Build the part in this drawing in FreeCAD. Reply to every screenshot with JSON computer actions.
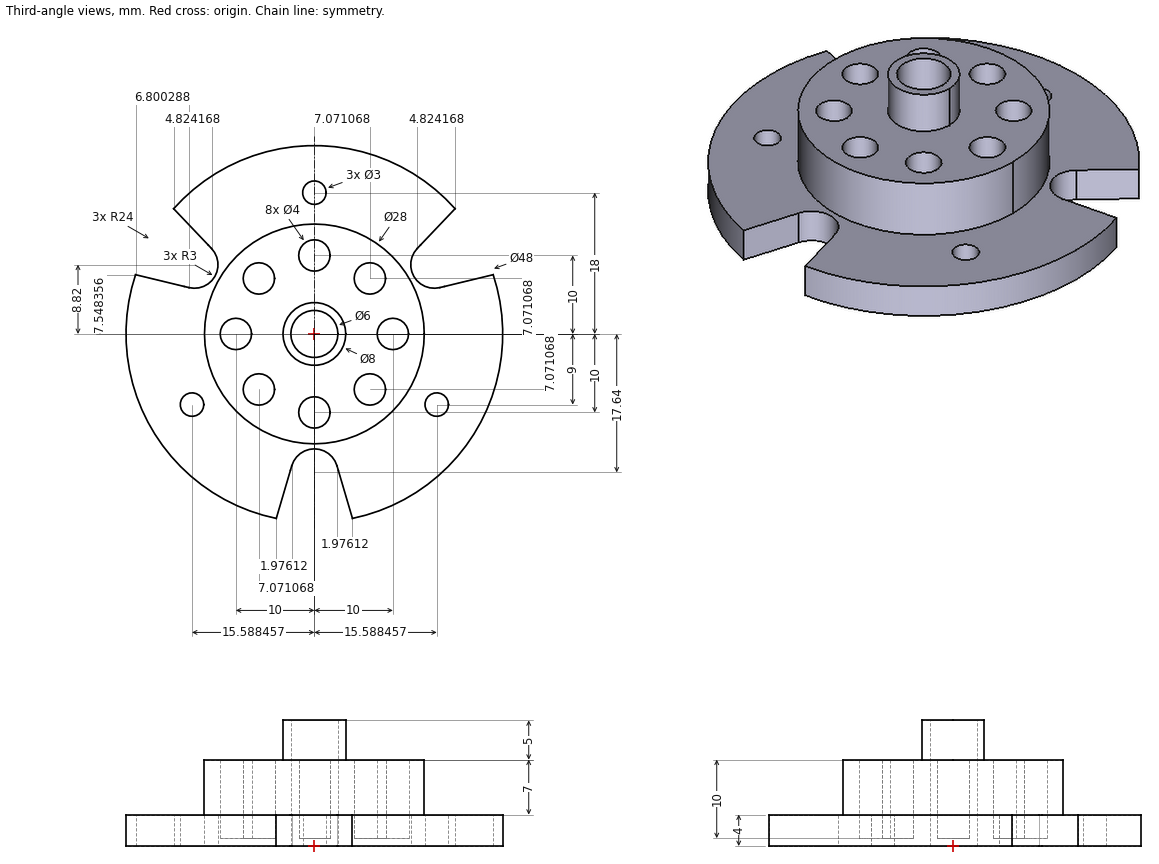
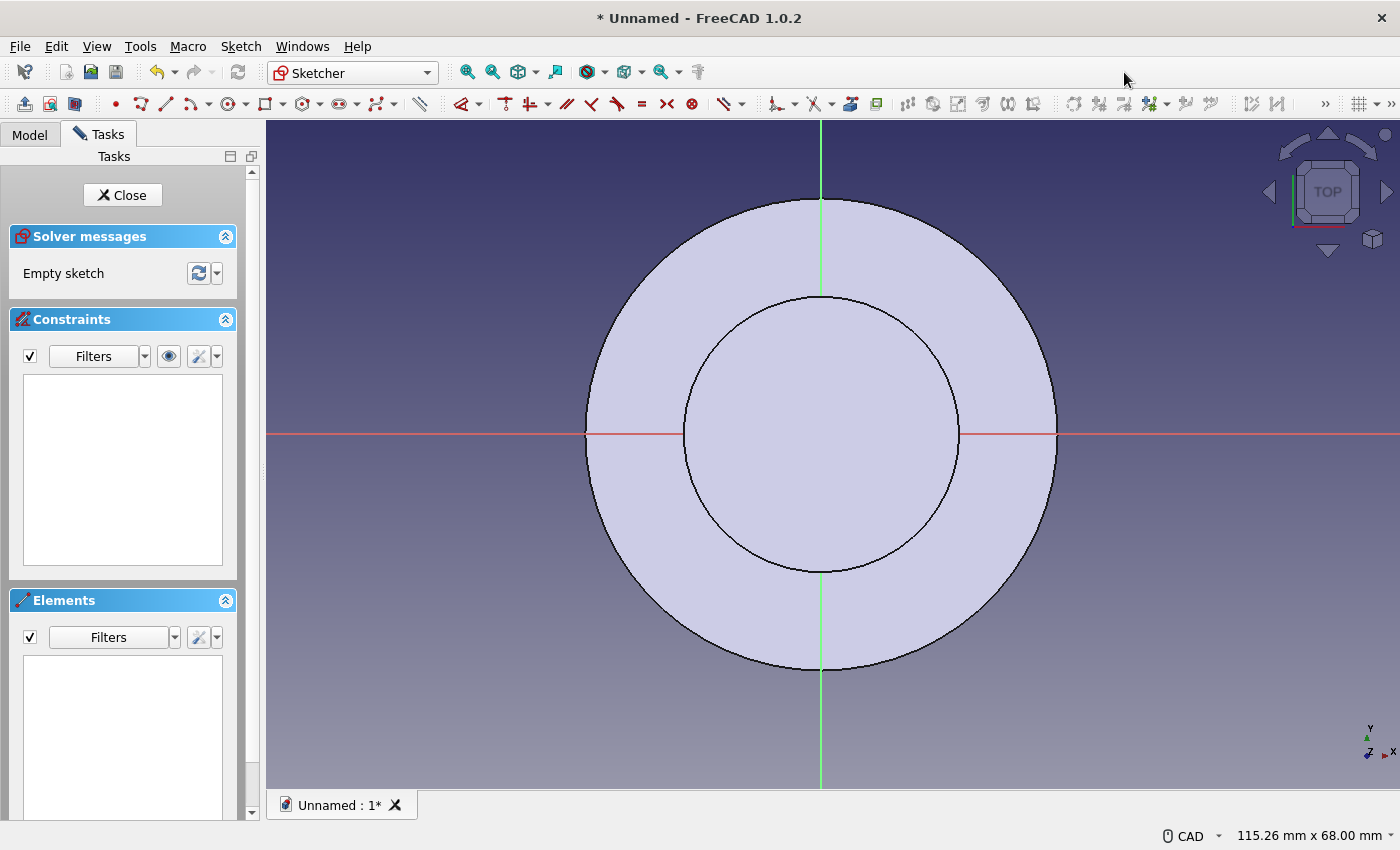
{"action": "left_click", "coordinate": [75, 104]}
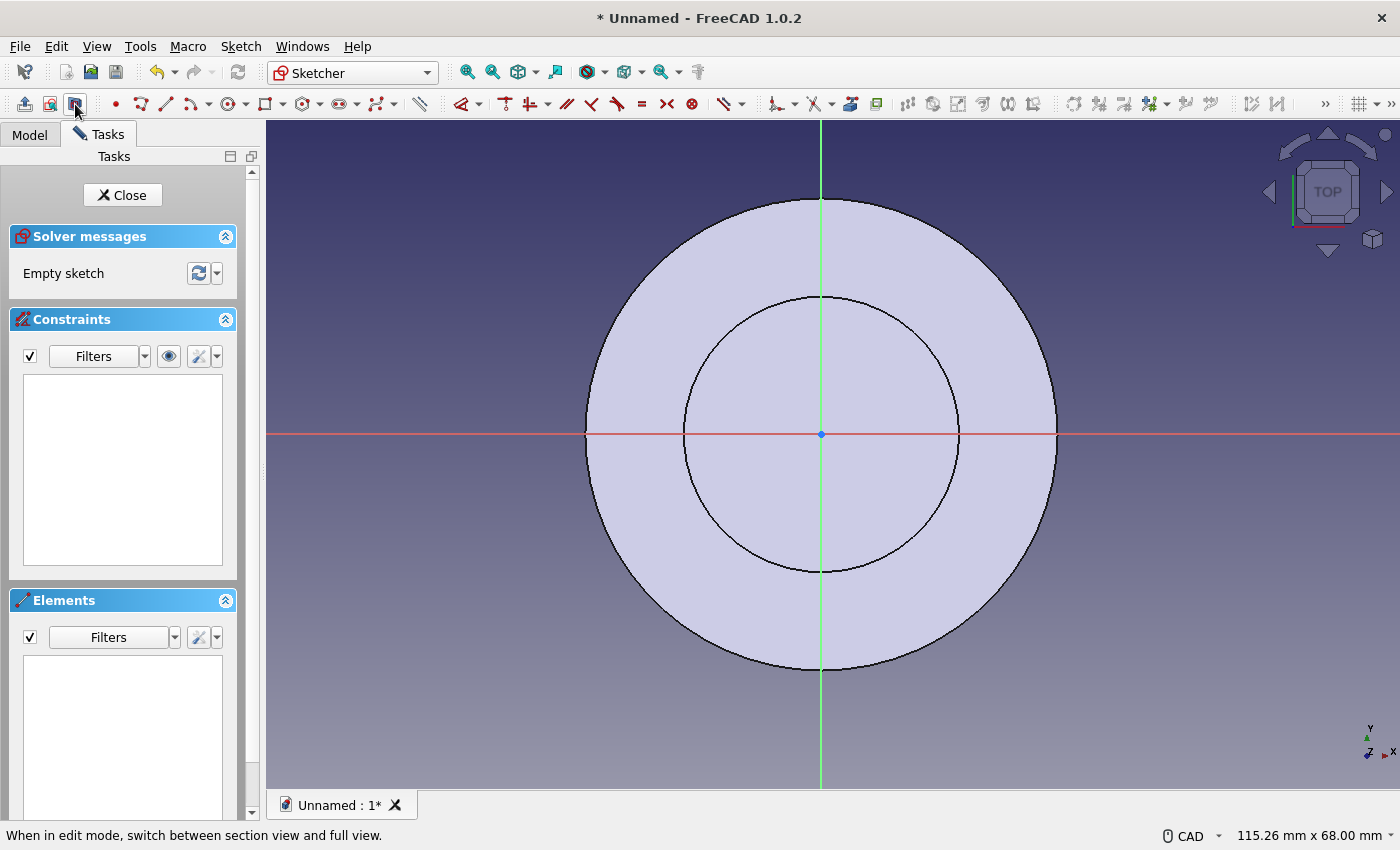
{"action": "scroll", "coordinate": [937, 259], "scroll_direction": "up", "scroll_amount": 2}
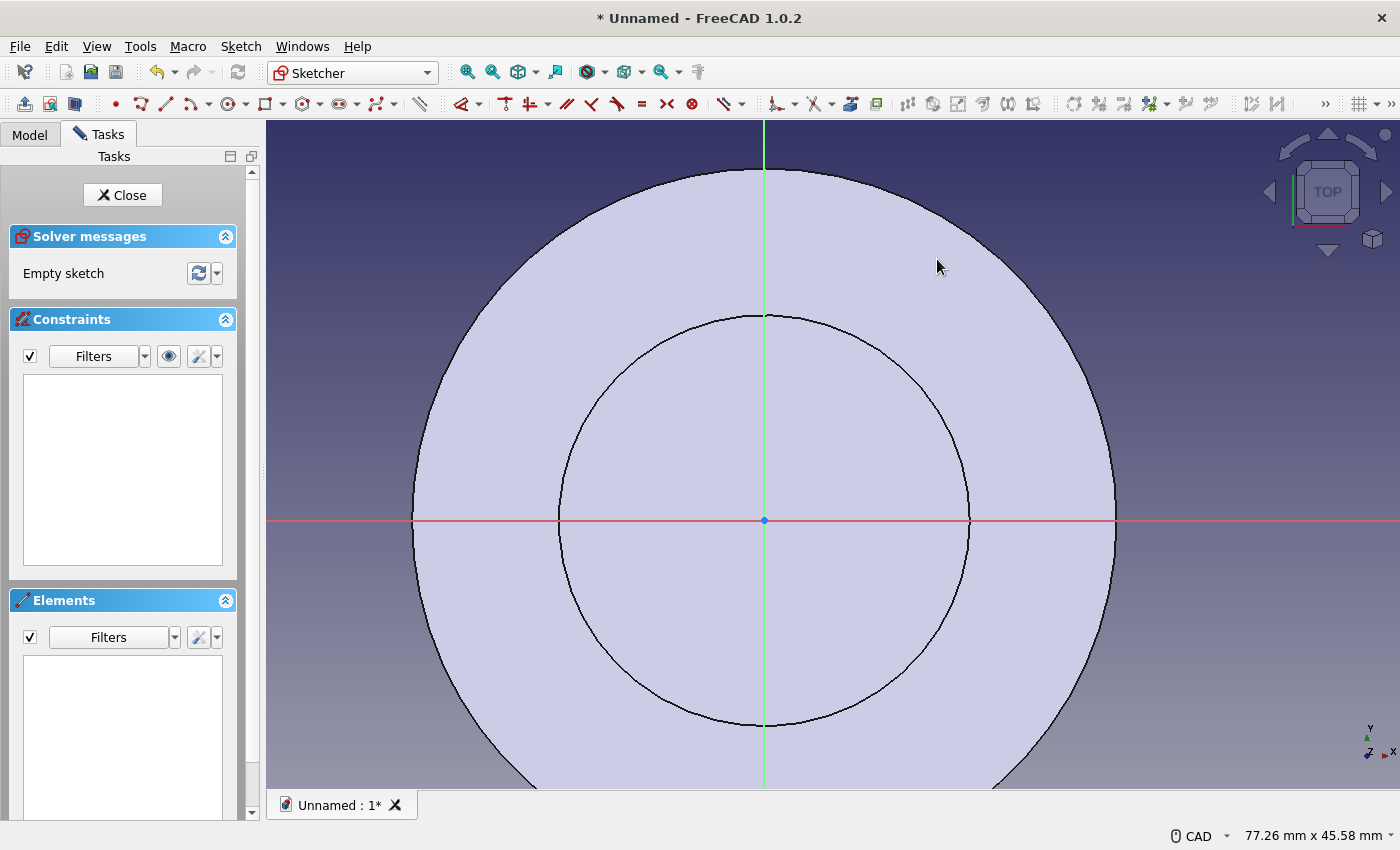
{"action": "left_click", "coordinate": [228, 104]}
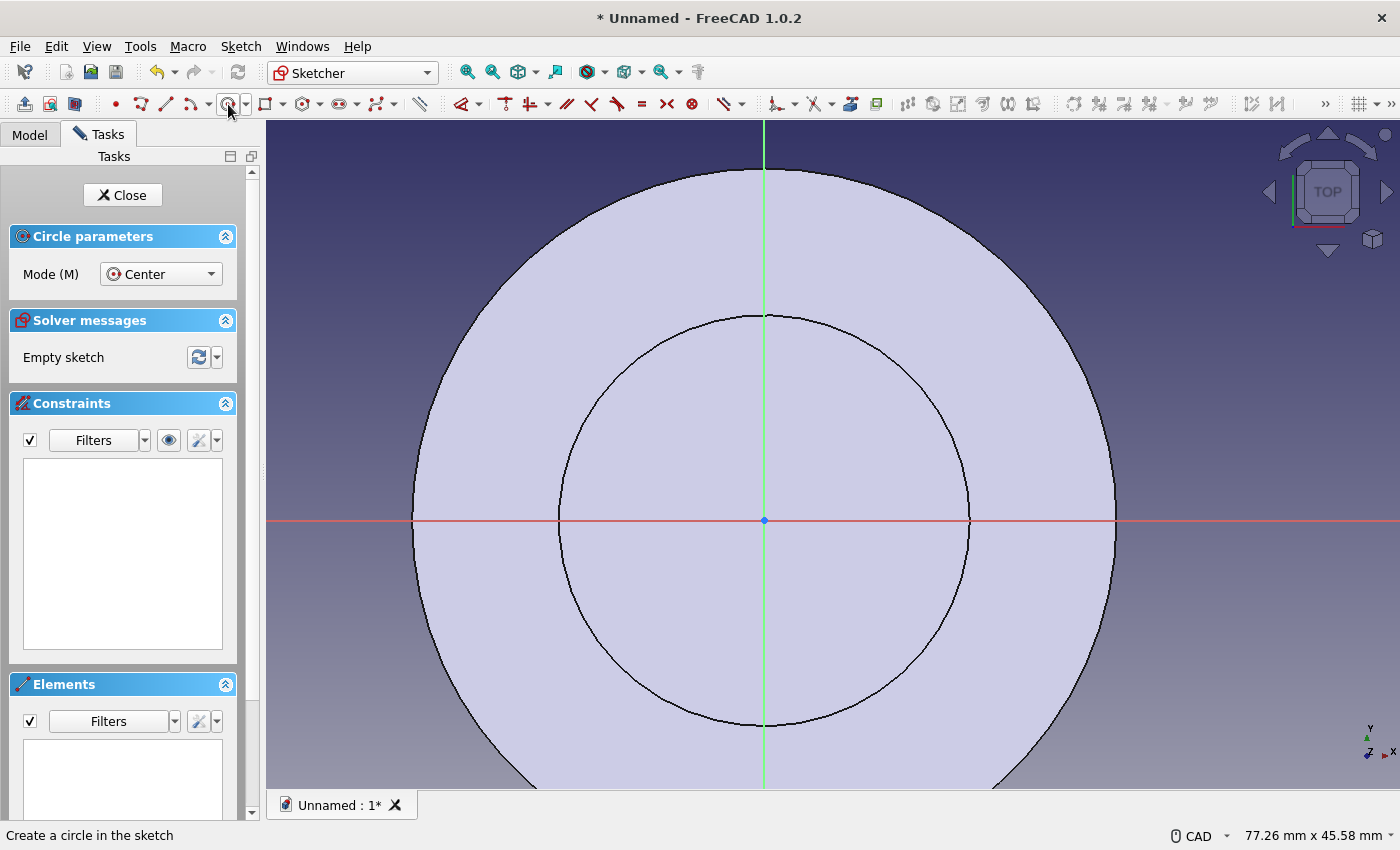
{"action": "left_click", "coordinate": [764, 256]}
{"action": "mouse_move", "coordinate": [780, 241]}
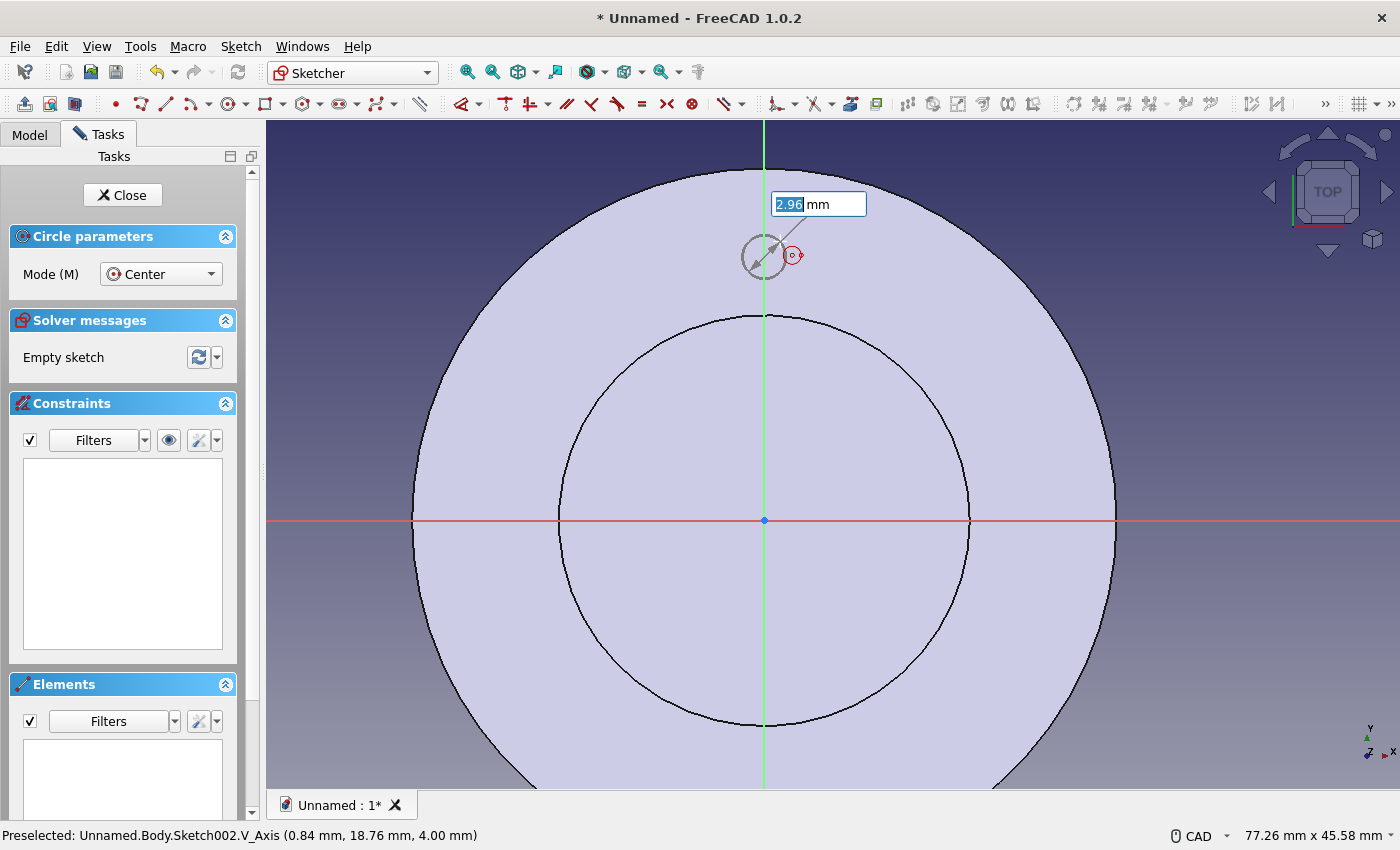
{"action": "type", "text": "3"}
{"action": "key", "text": "Return"}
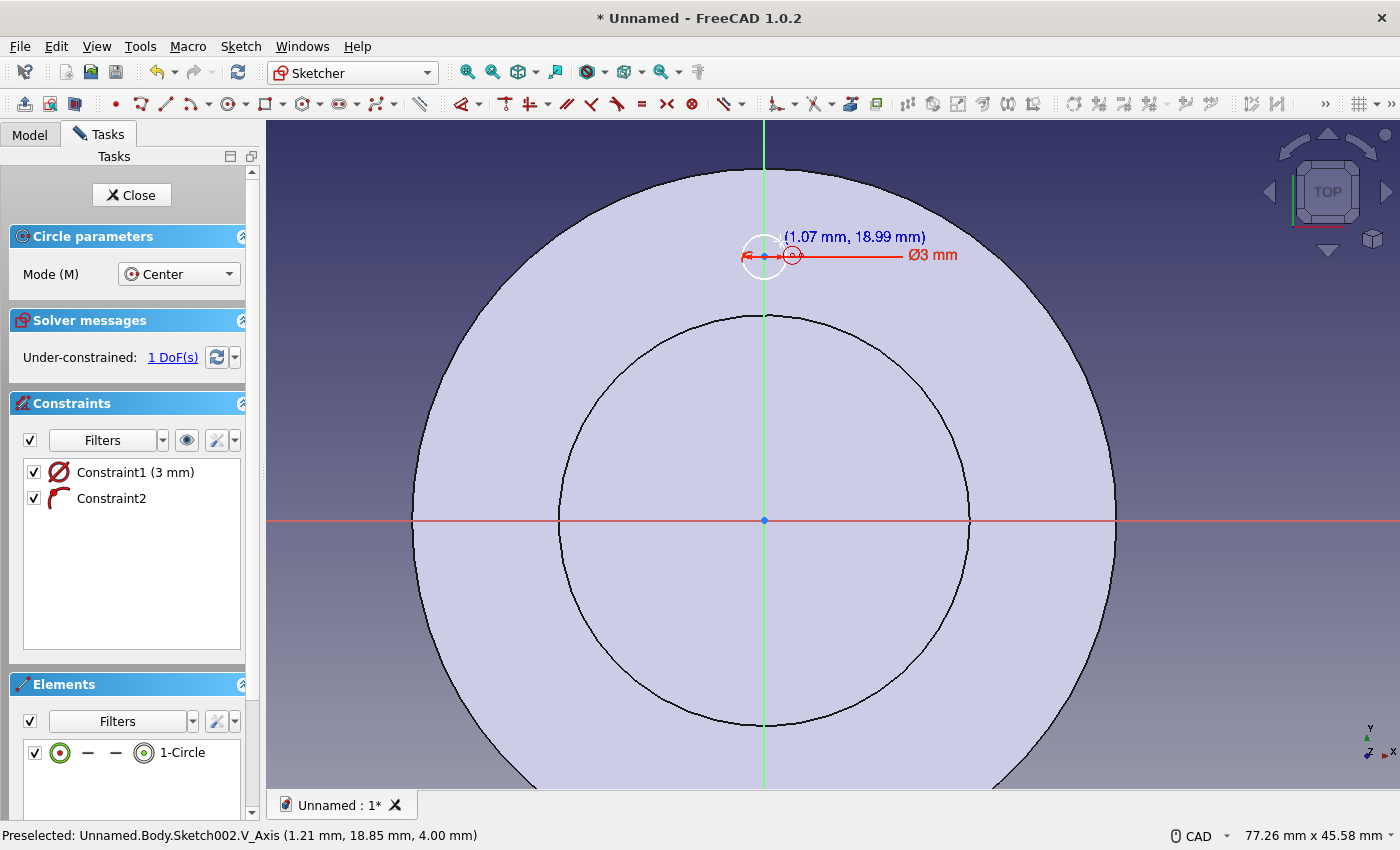
{"action": "left_click", "coordinate": [993, 653]}
{"action": "mouse_move", "coordinate": [1009, 637]}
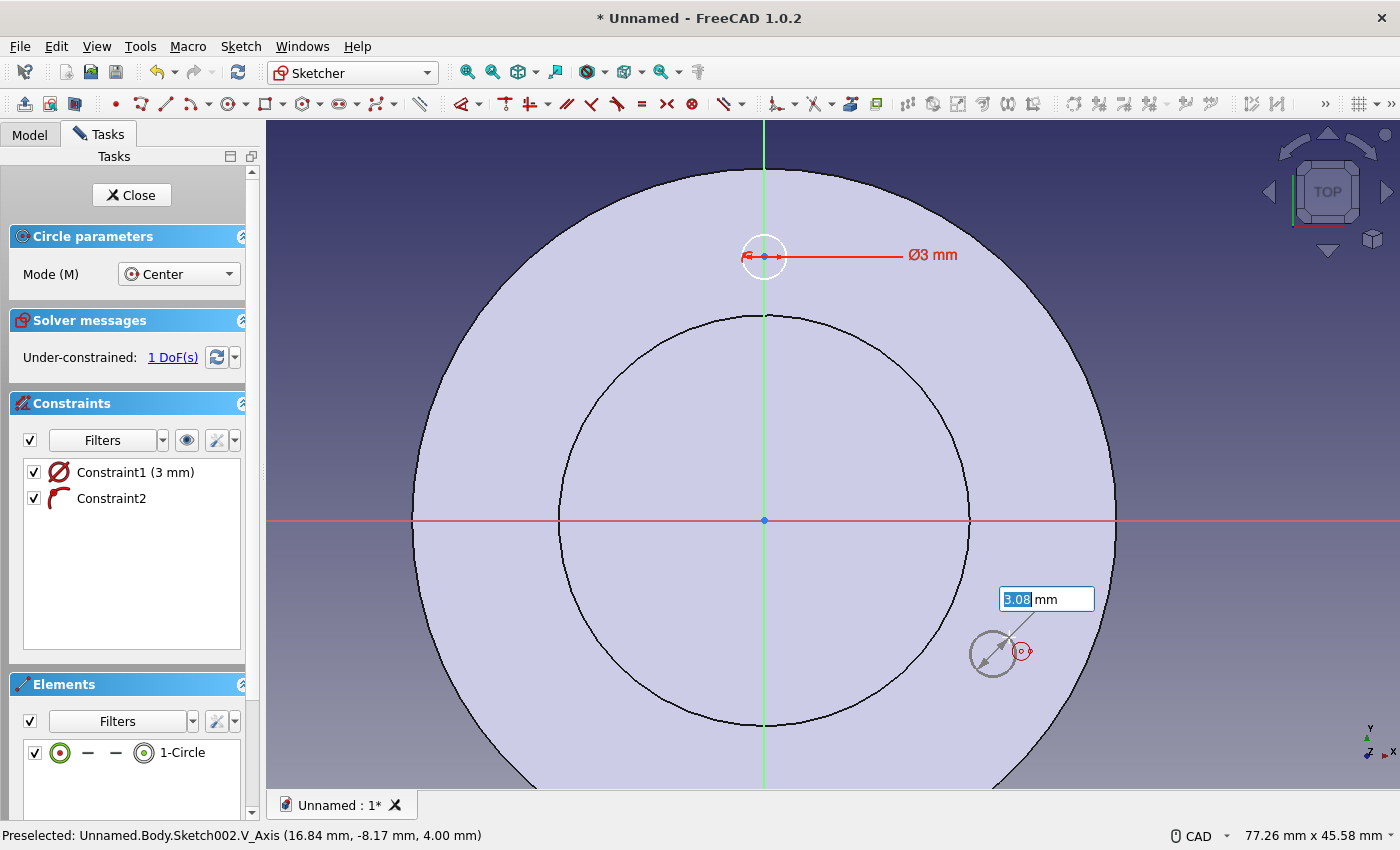
{"action": "type", "text": "3"}
{"action": "key", "text": "Return"}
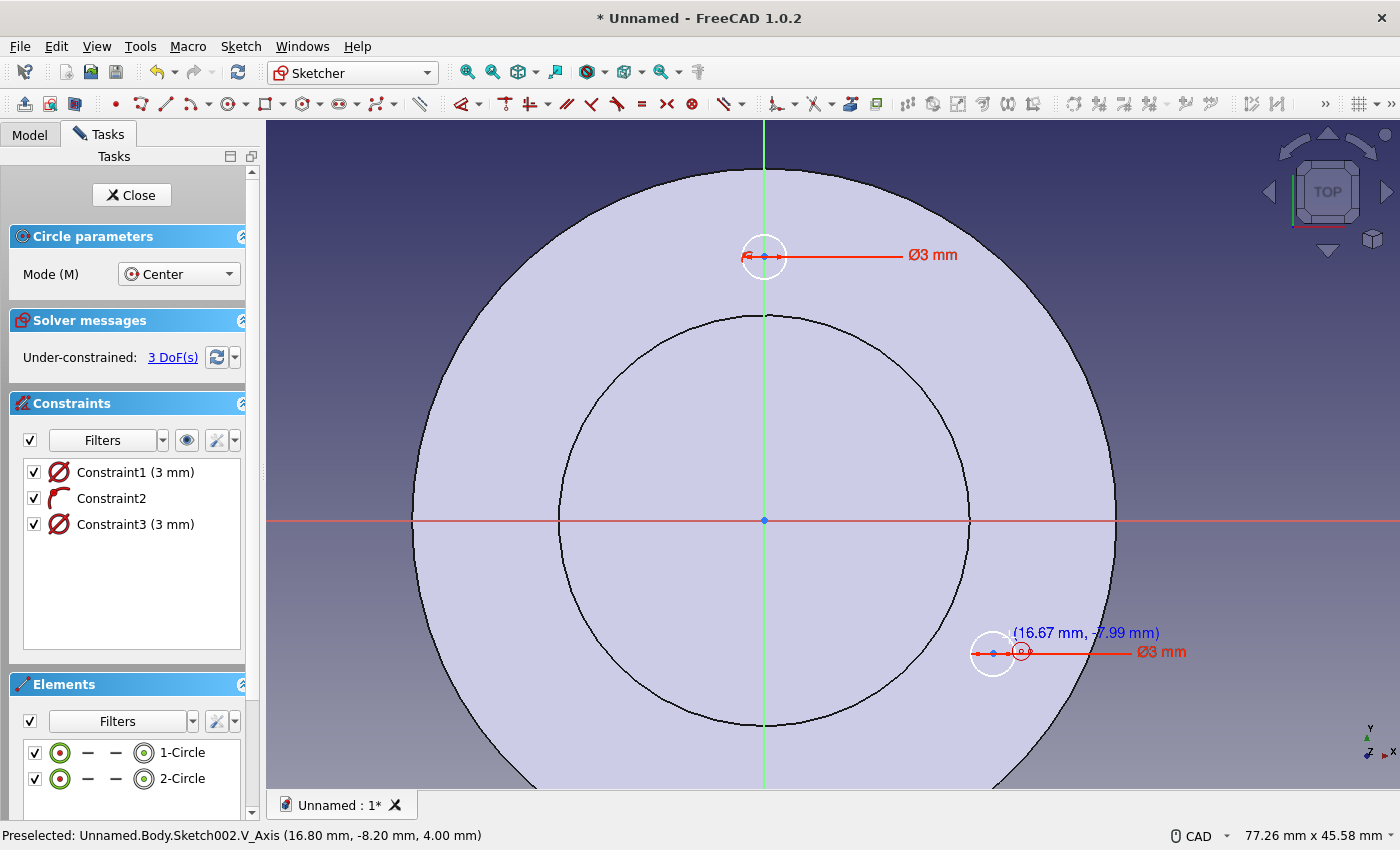
{"action": "left_click", "coordinate": [536, 653]}
{"action": "mouse_move", "coordinate": [551, 637]}